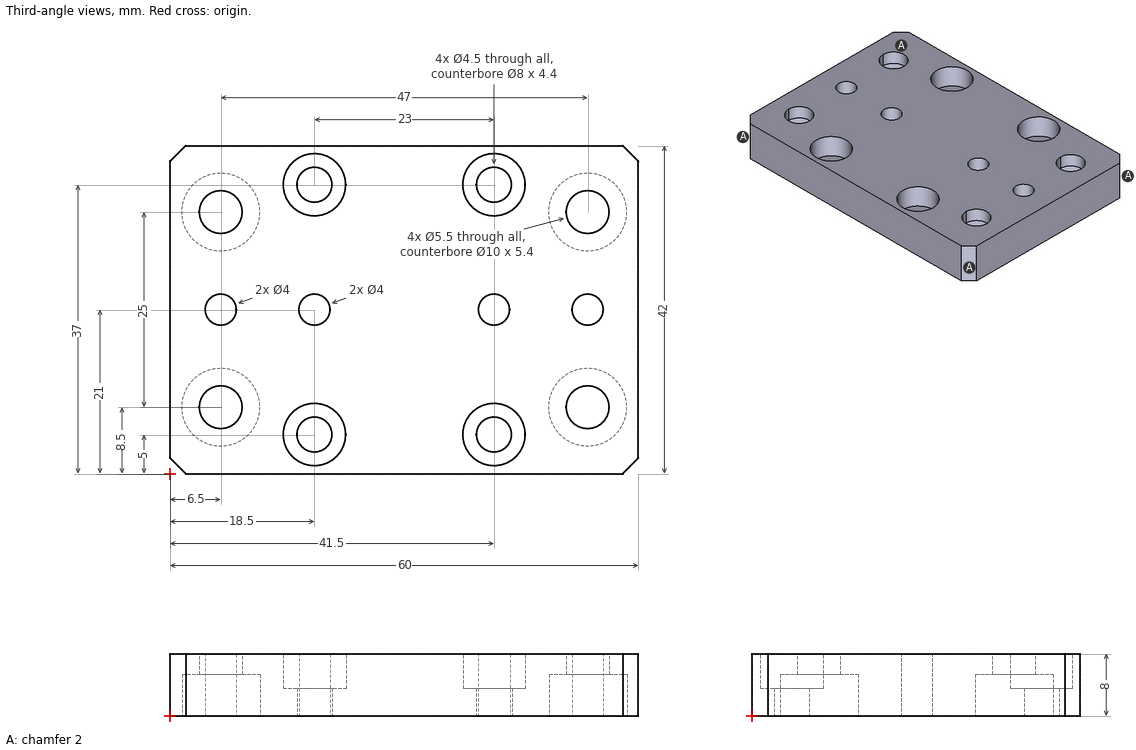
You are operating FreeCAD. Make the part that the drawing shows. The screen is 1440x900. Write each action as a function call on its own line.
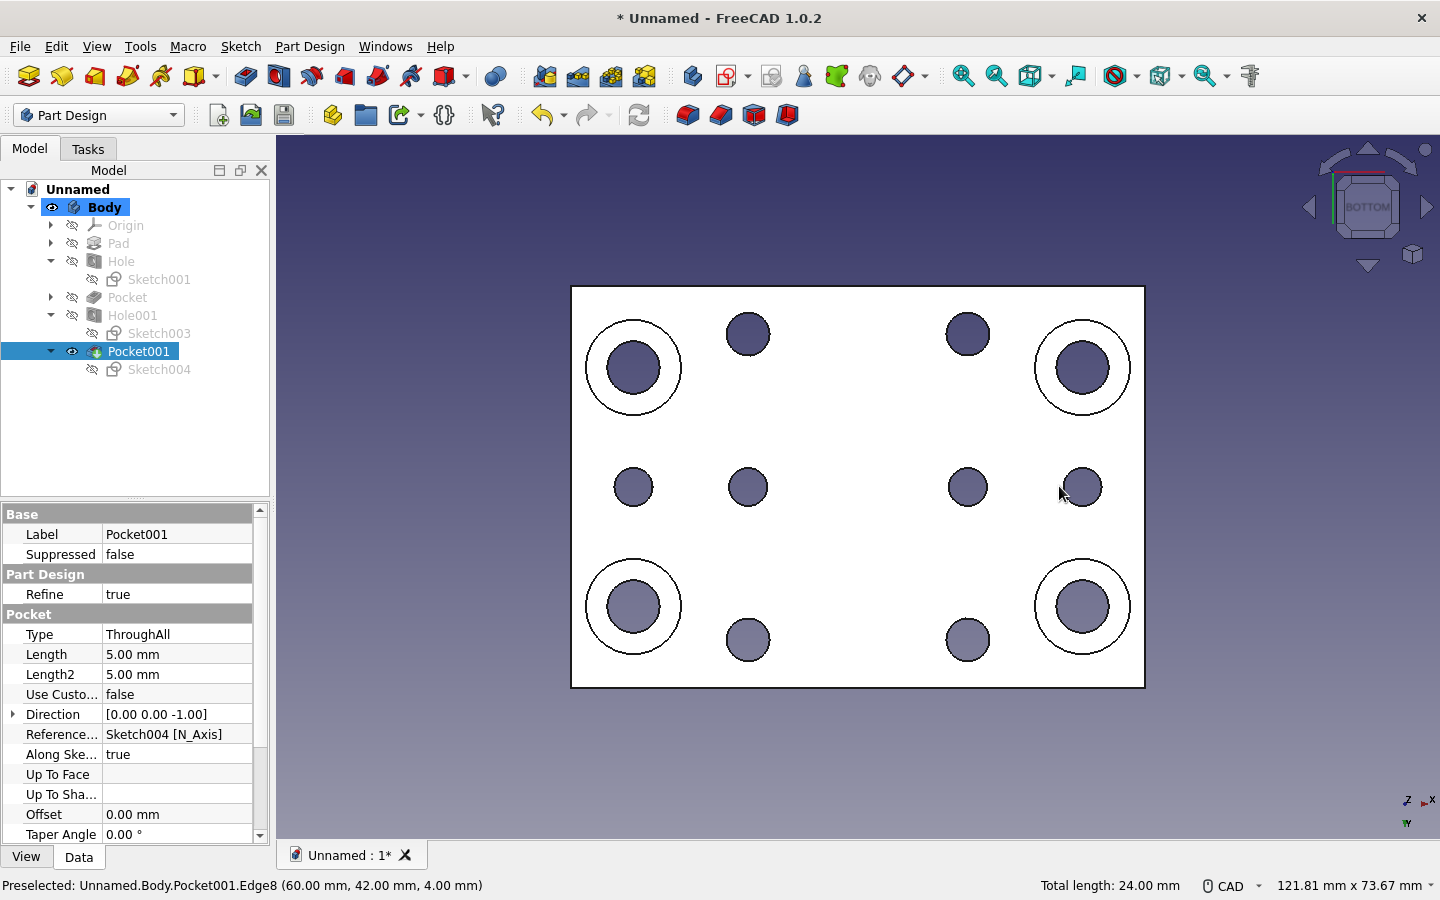
key(4)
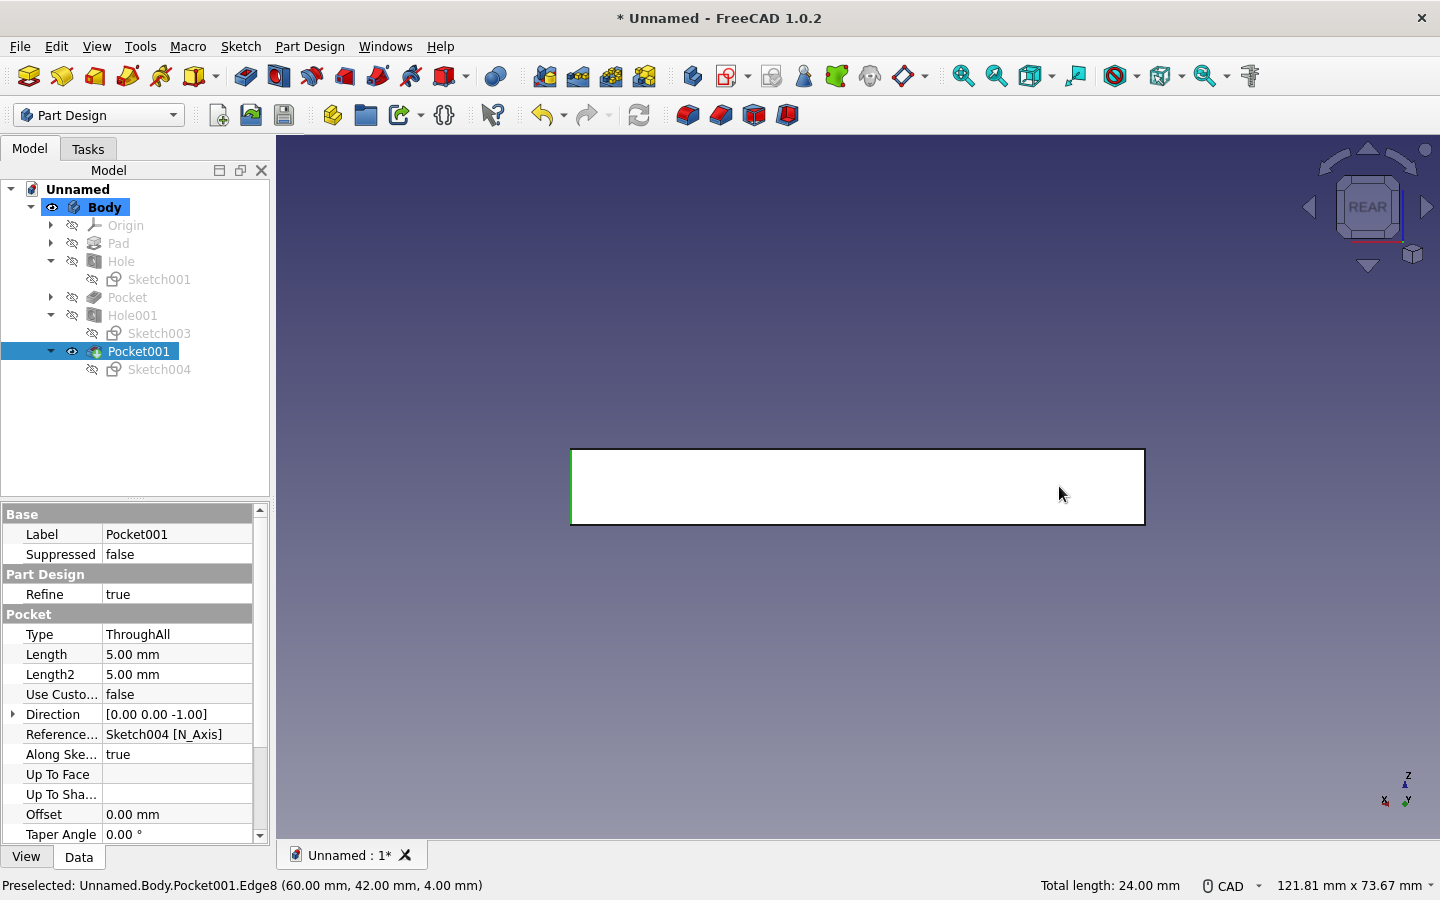
click(1145, 486, ctrl)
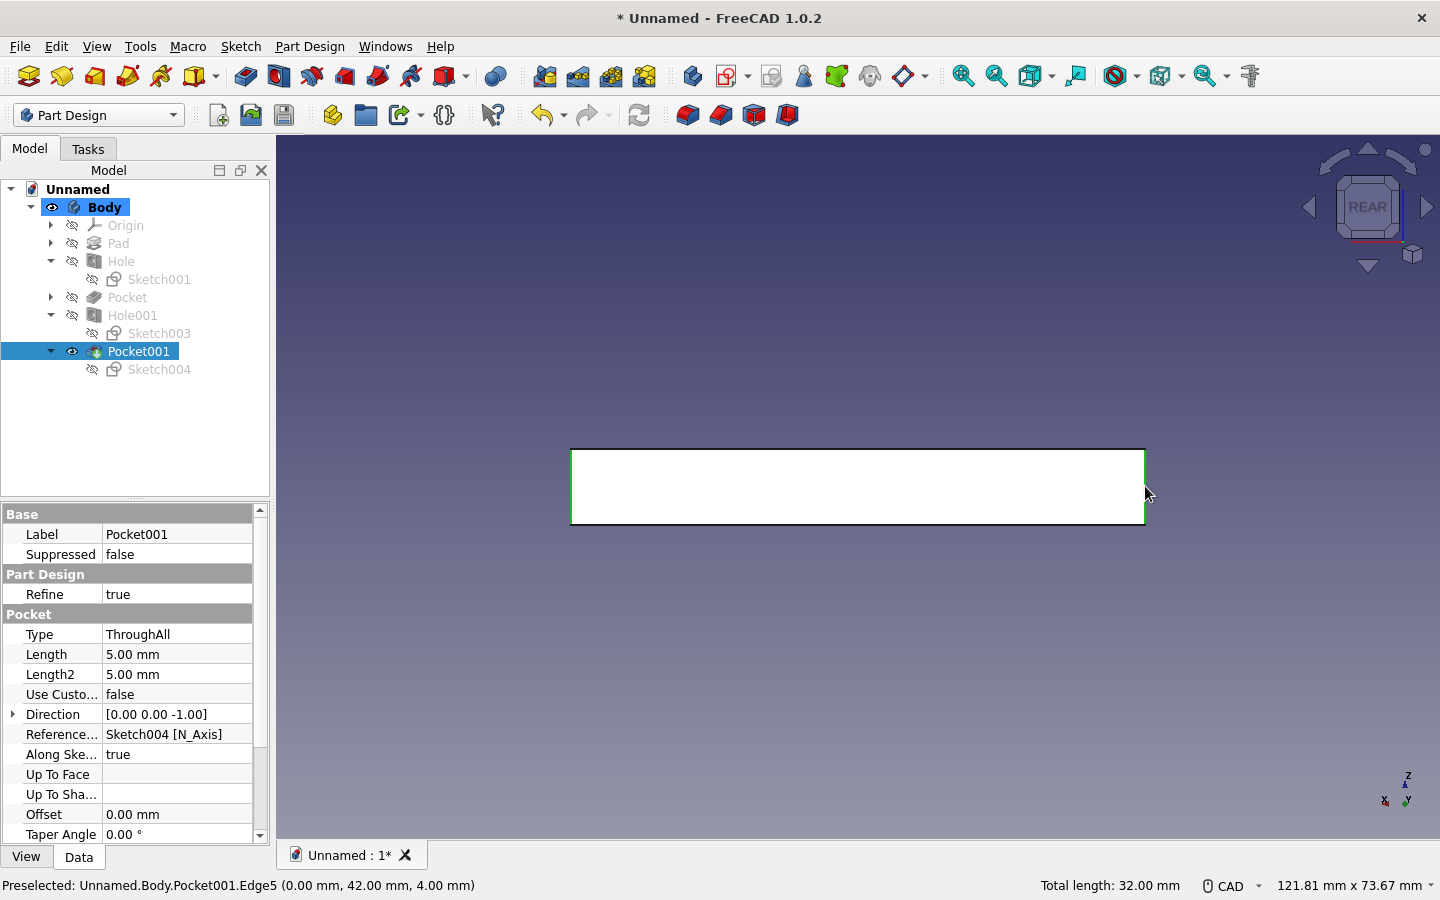
click(721, 116)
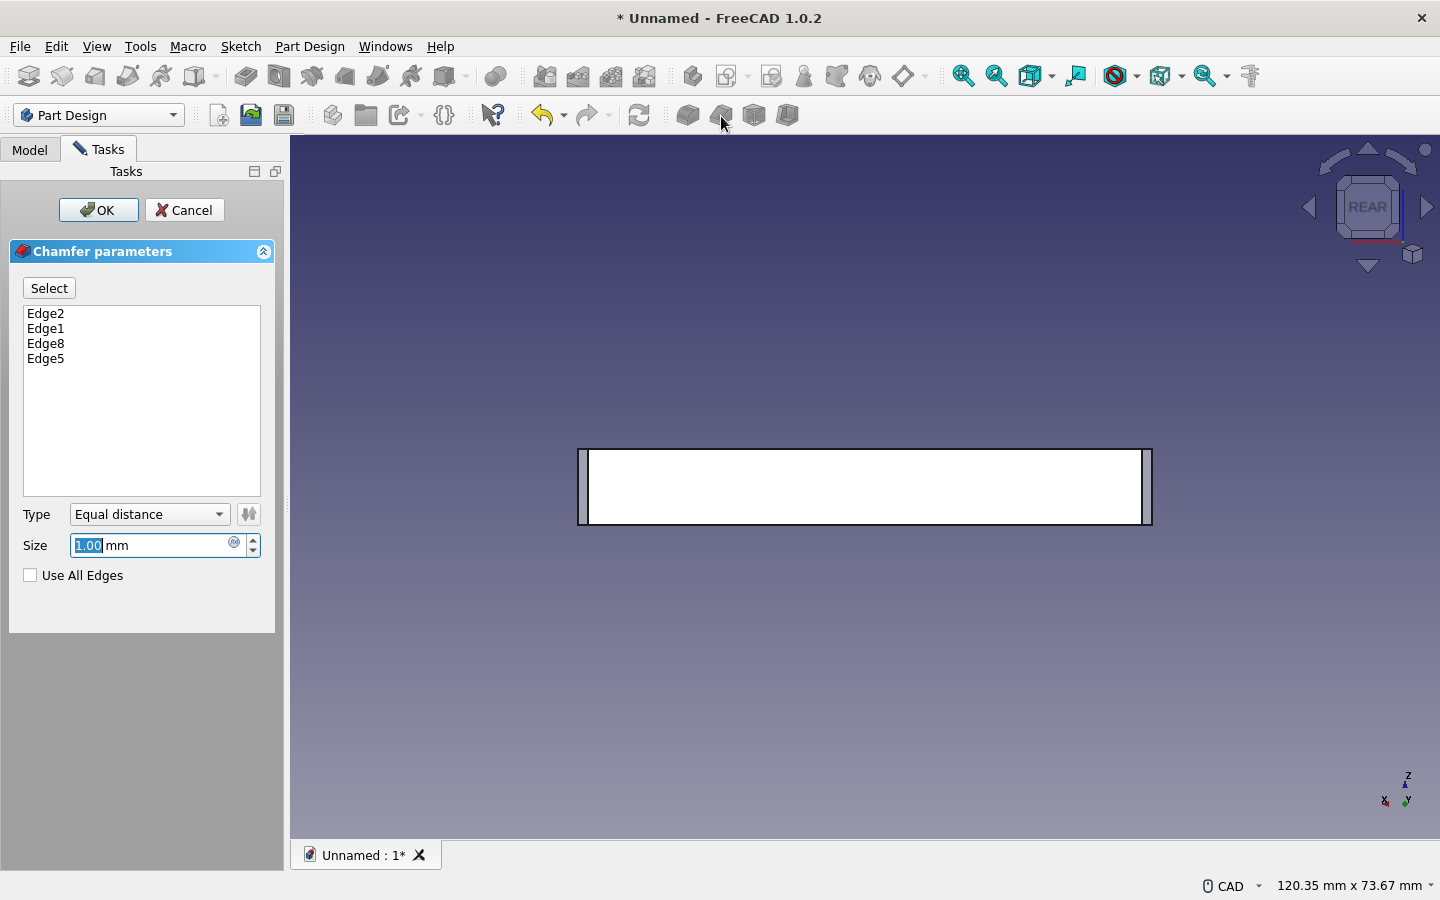
text(2)
key(Tab)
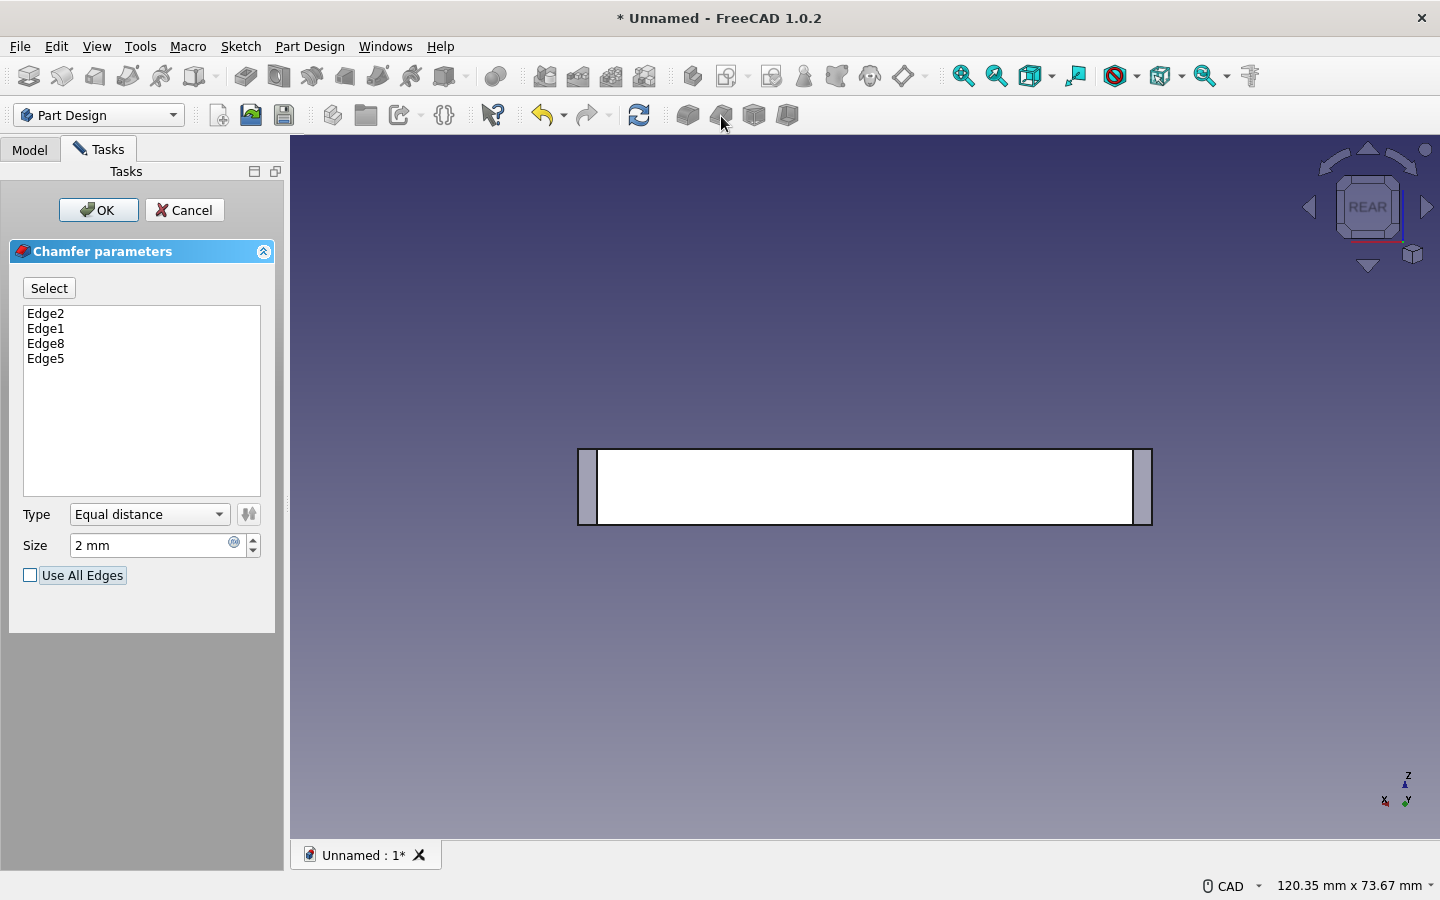
click(99, 210)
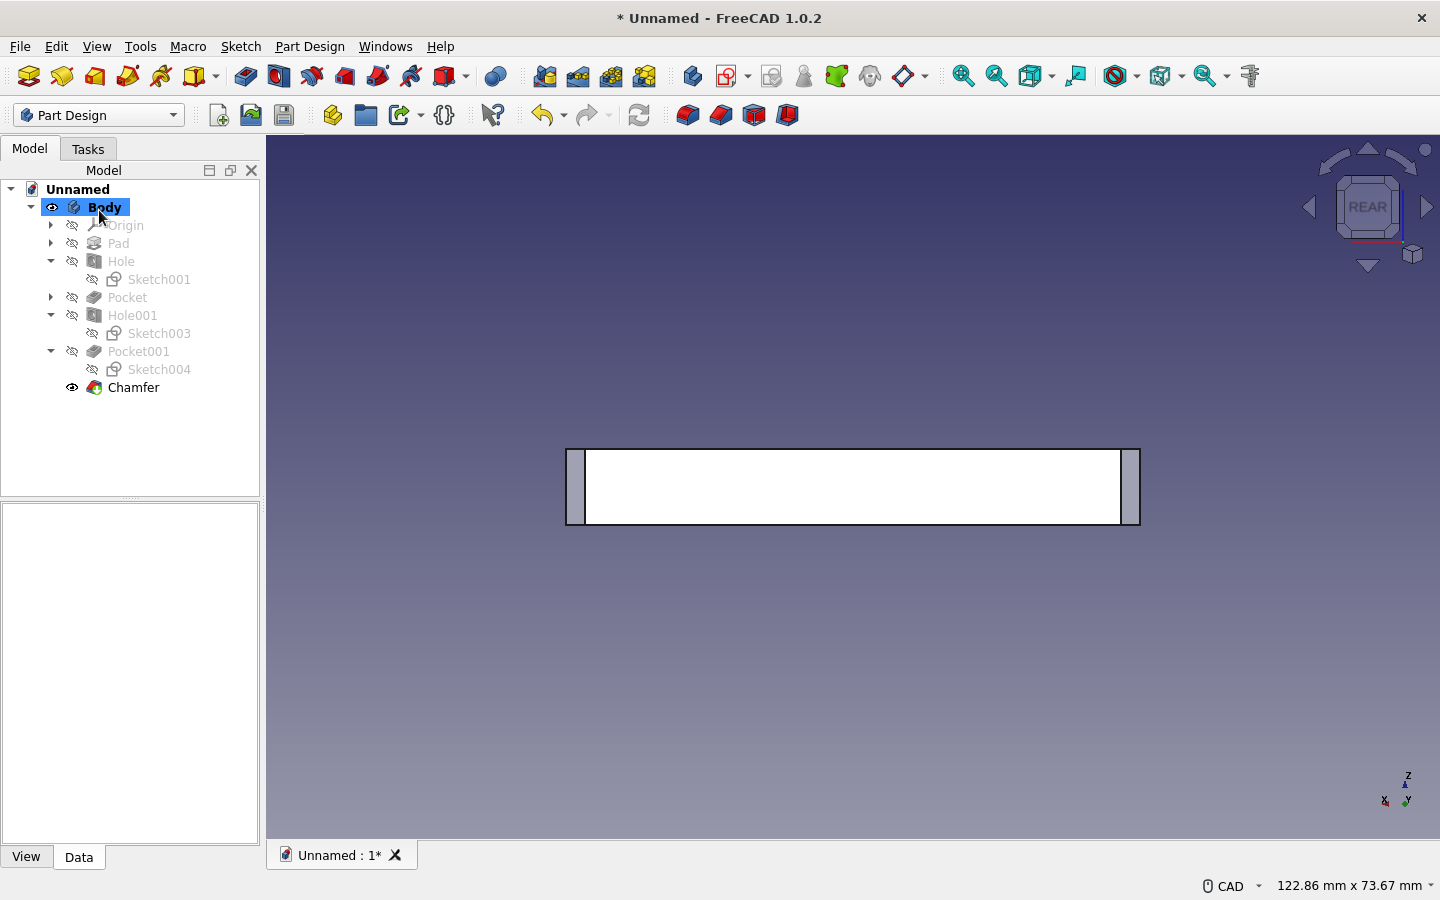
key(0)